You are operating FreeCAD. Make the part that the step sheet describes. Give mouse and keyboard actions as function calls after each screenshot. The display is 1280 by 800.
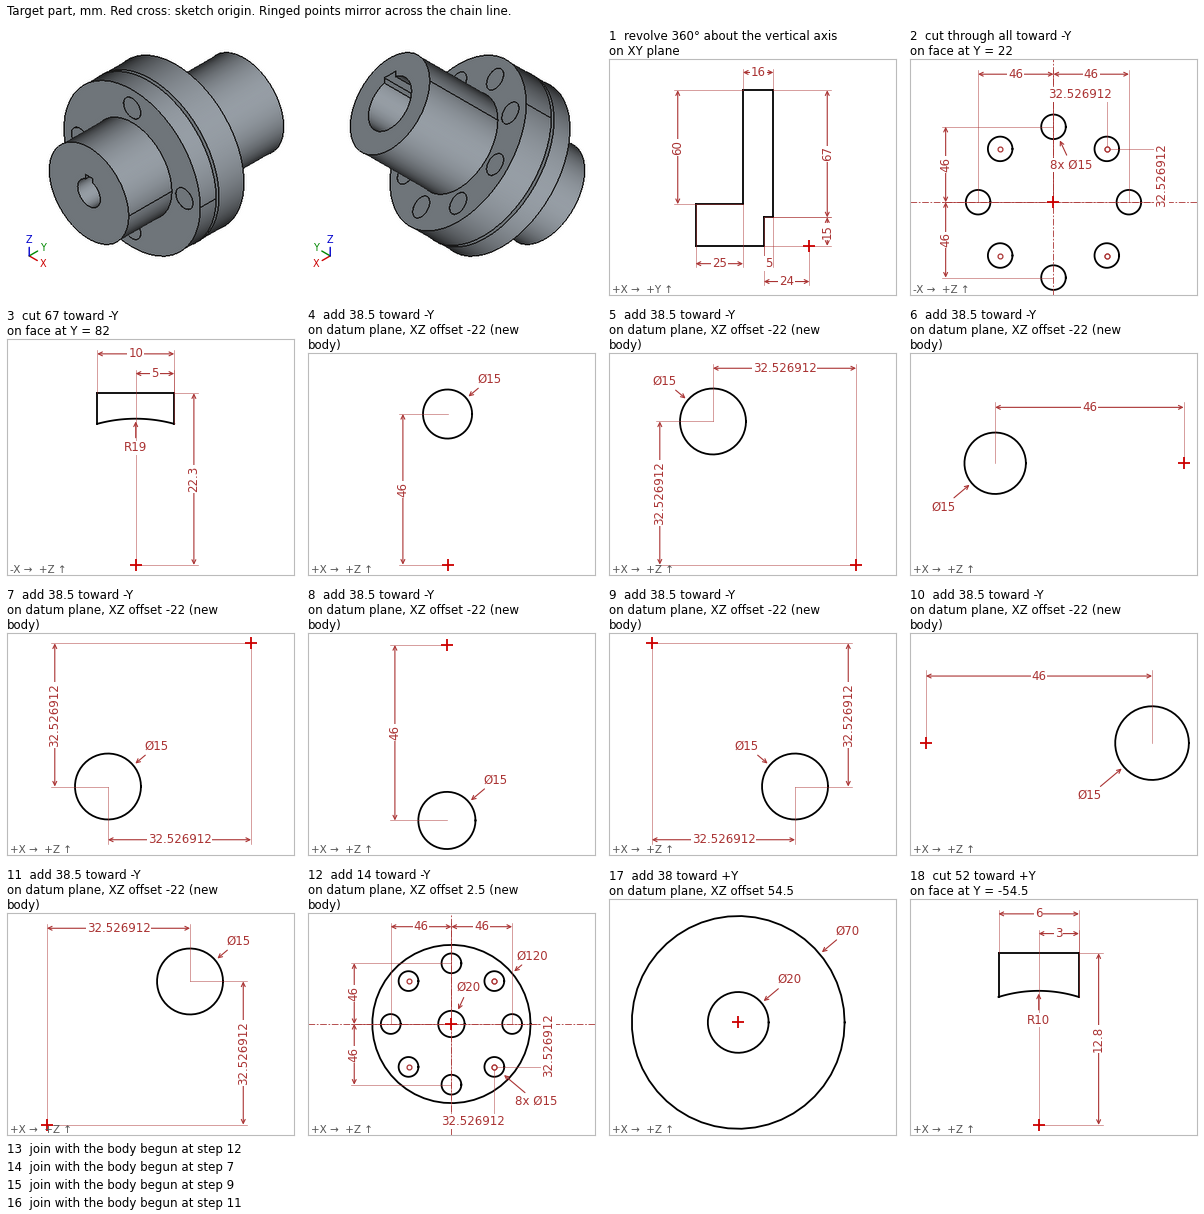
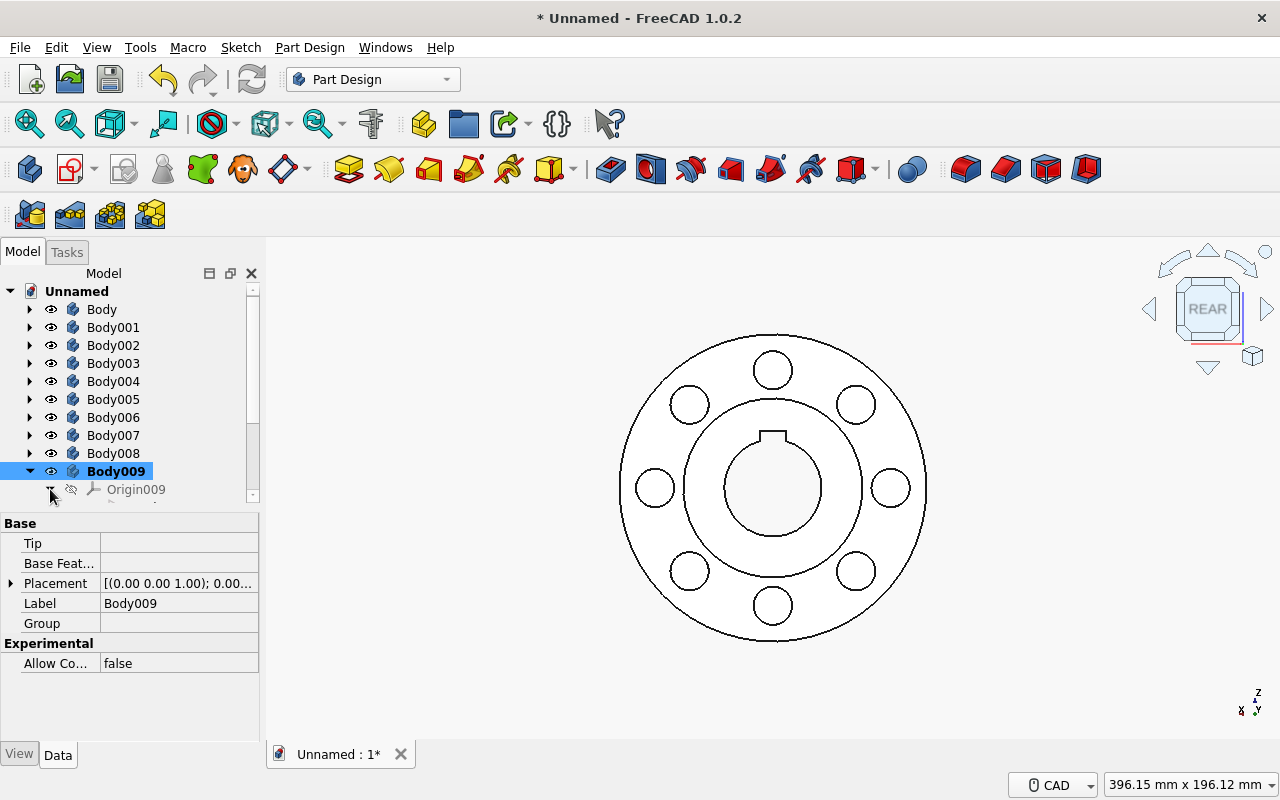
scroll(100, 395, down, 3)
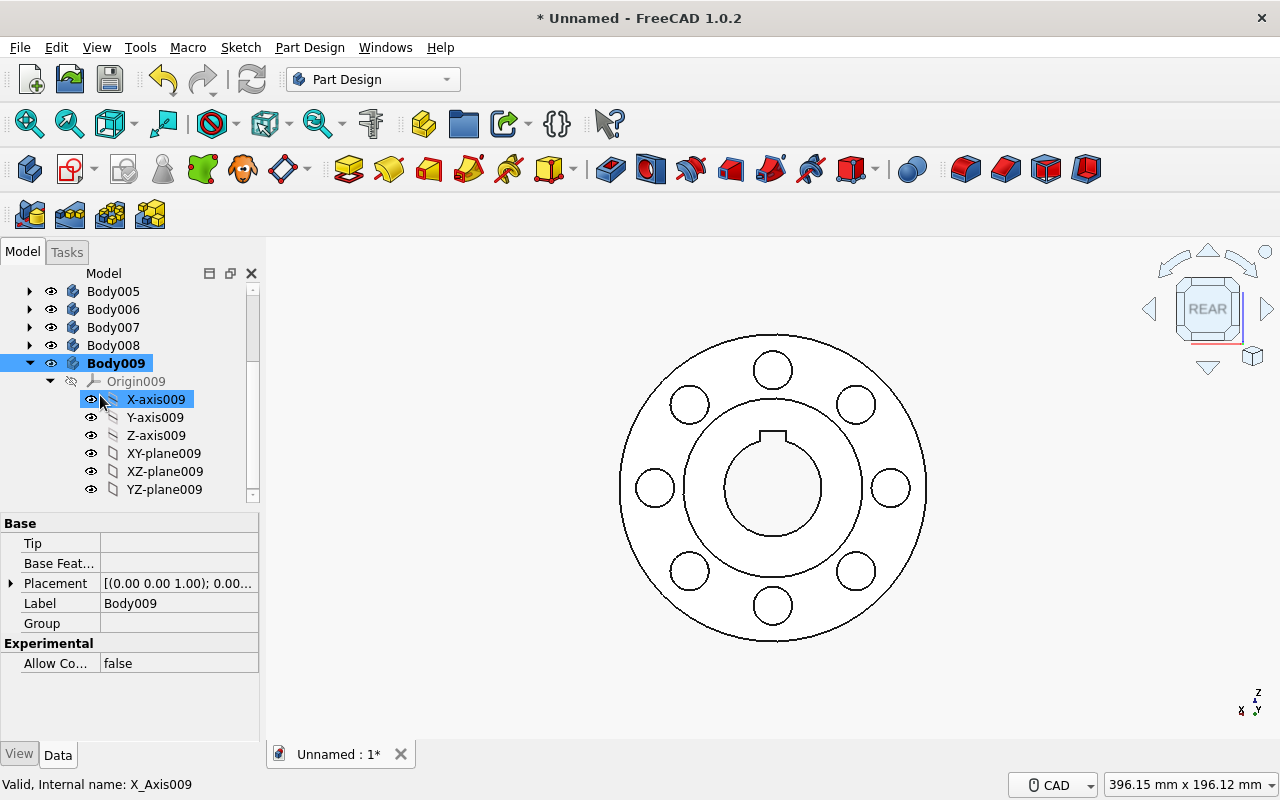
click(136, 471)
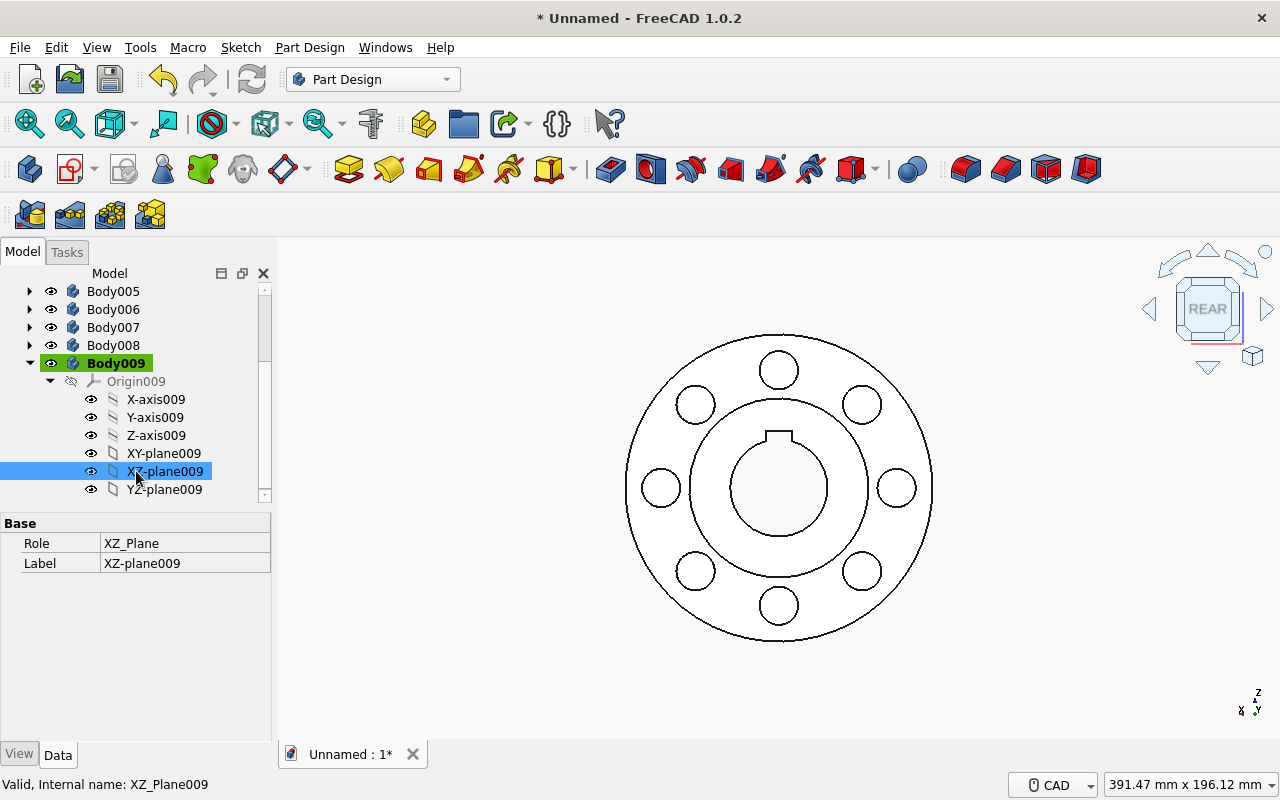
click(284, 170)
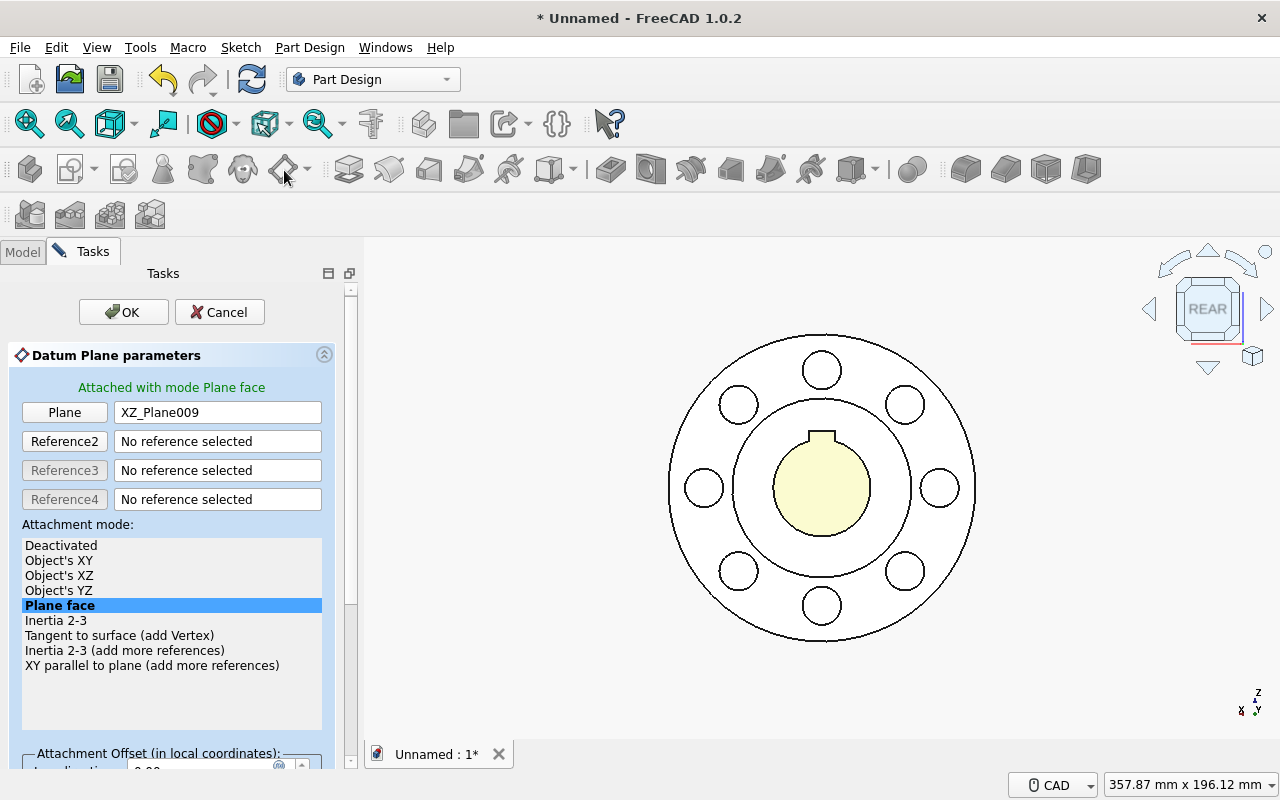
scroll(351, 526, down, 3)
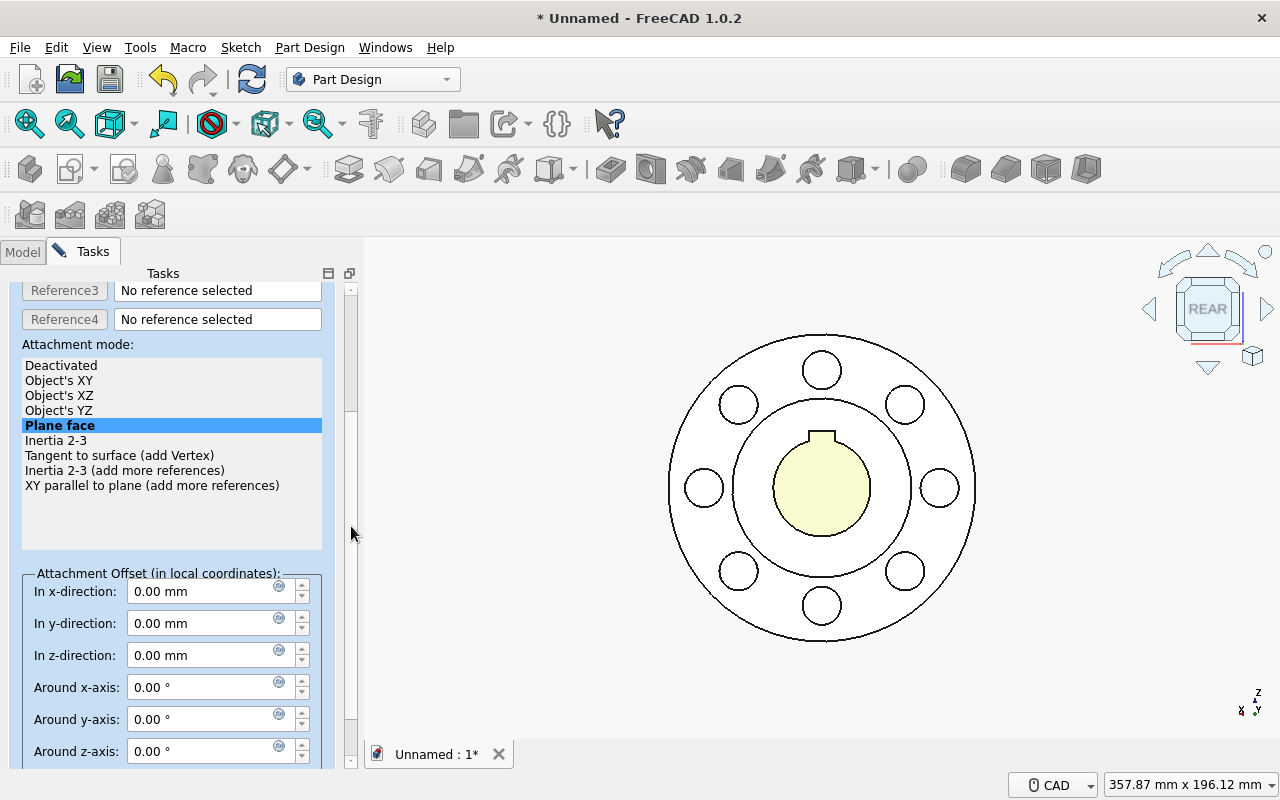
triple_click(210, 655)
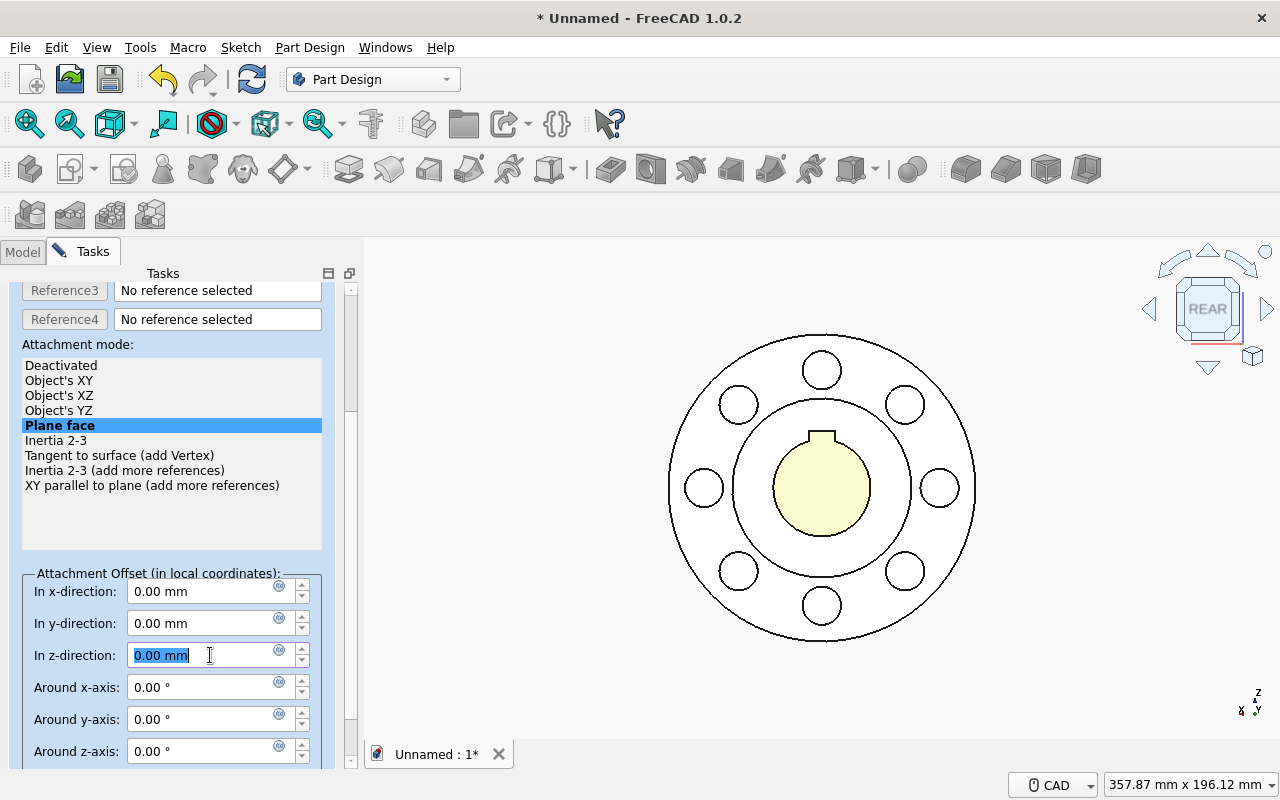
text(2.5)
key(Tab)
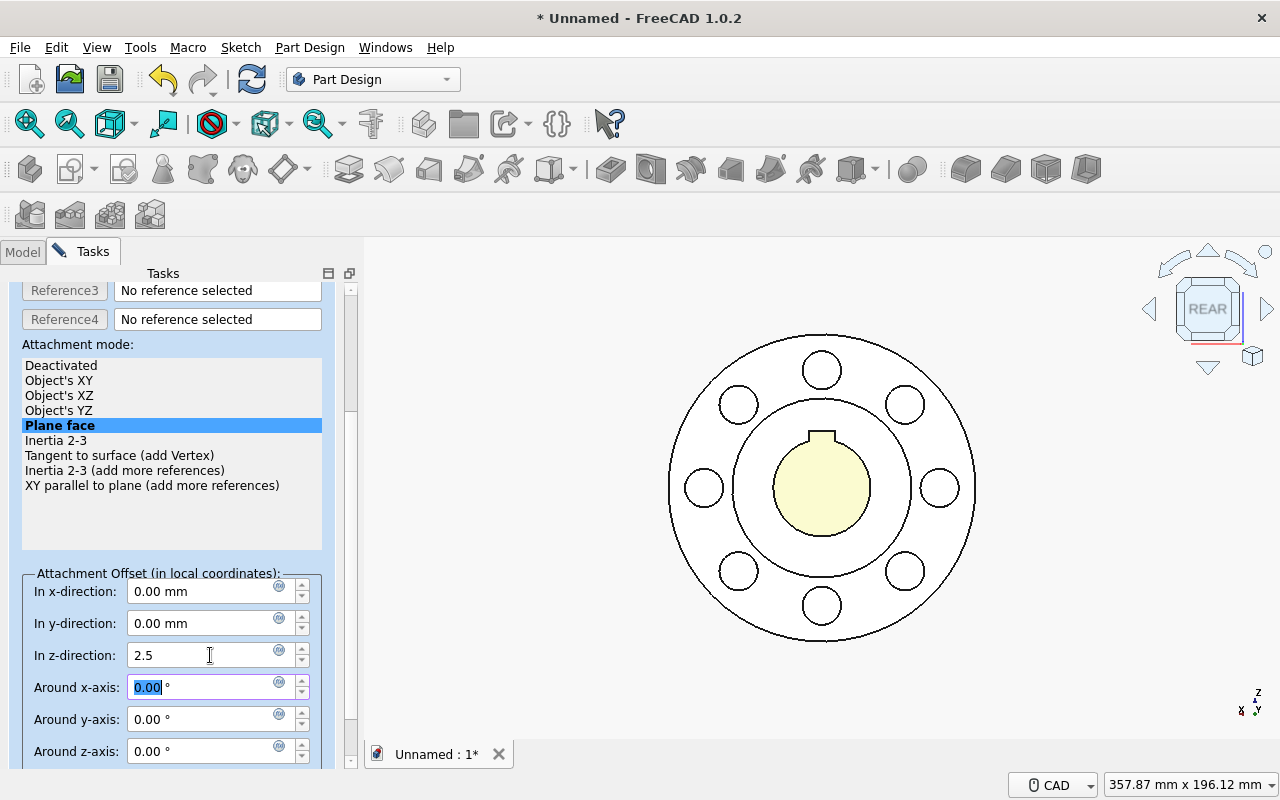
scroll(351, 526, up, 4)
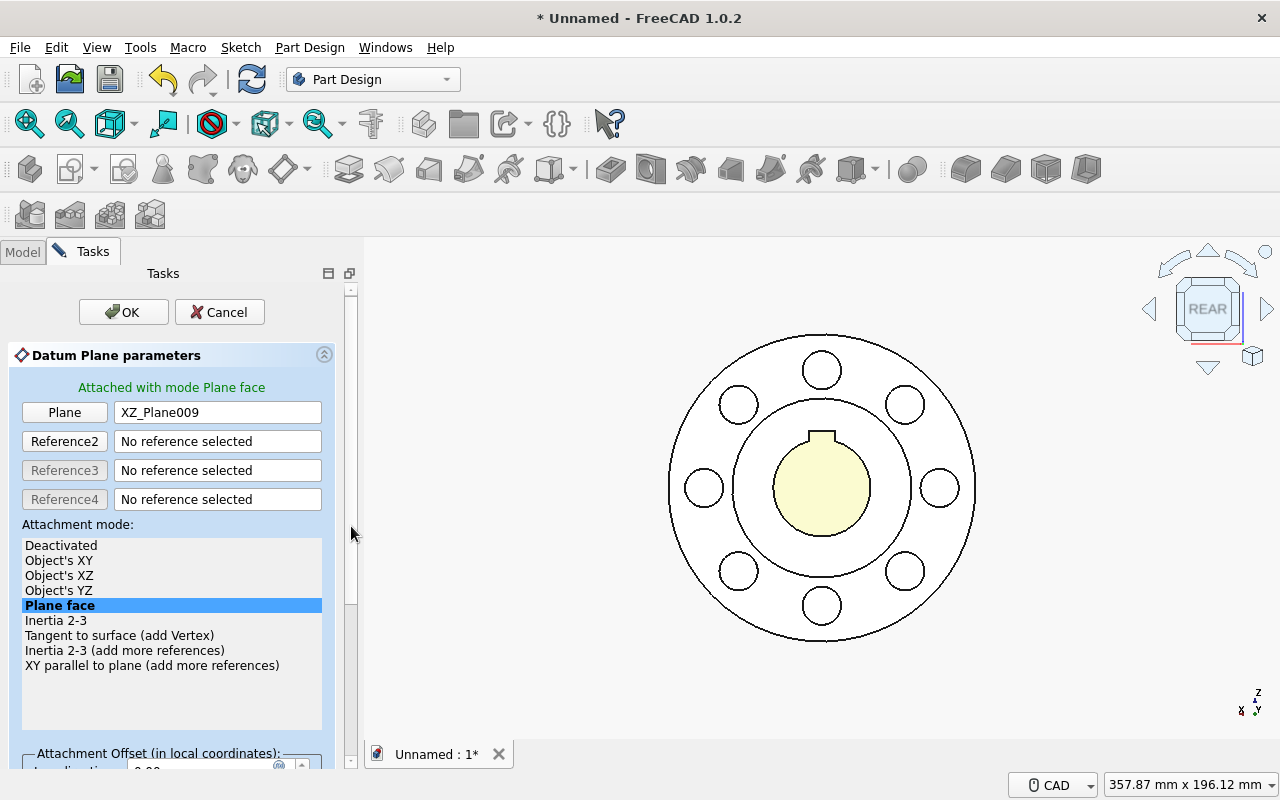
click(124, 312)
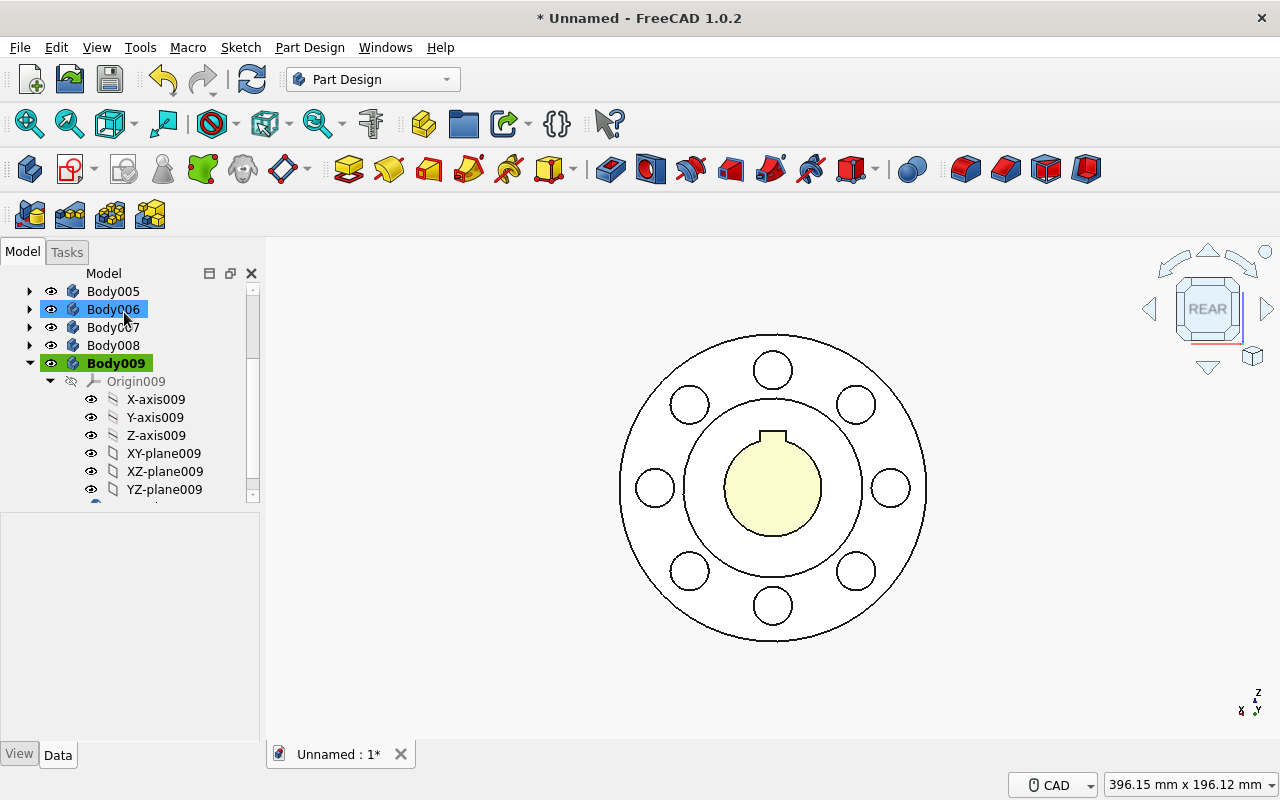
scroll(120, 395, down, 3)